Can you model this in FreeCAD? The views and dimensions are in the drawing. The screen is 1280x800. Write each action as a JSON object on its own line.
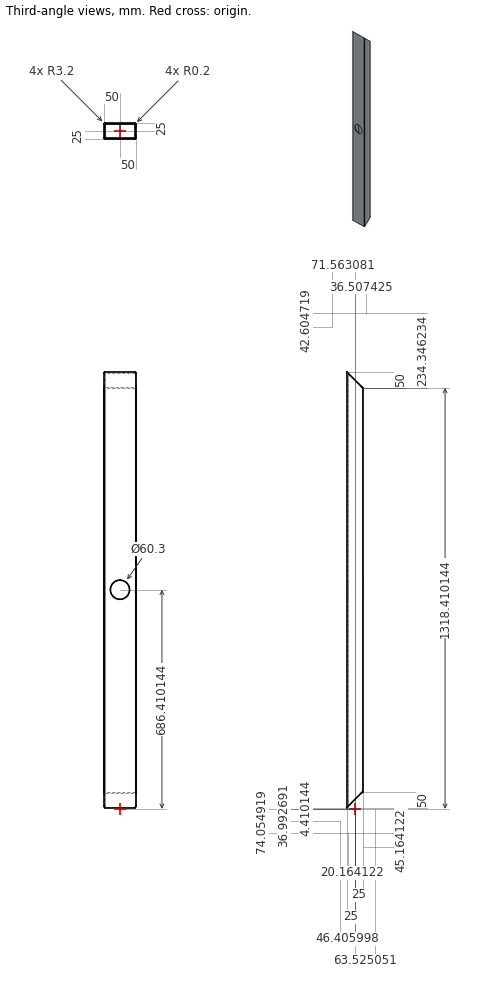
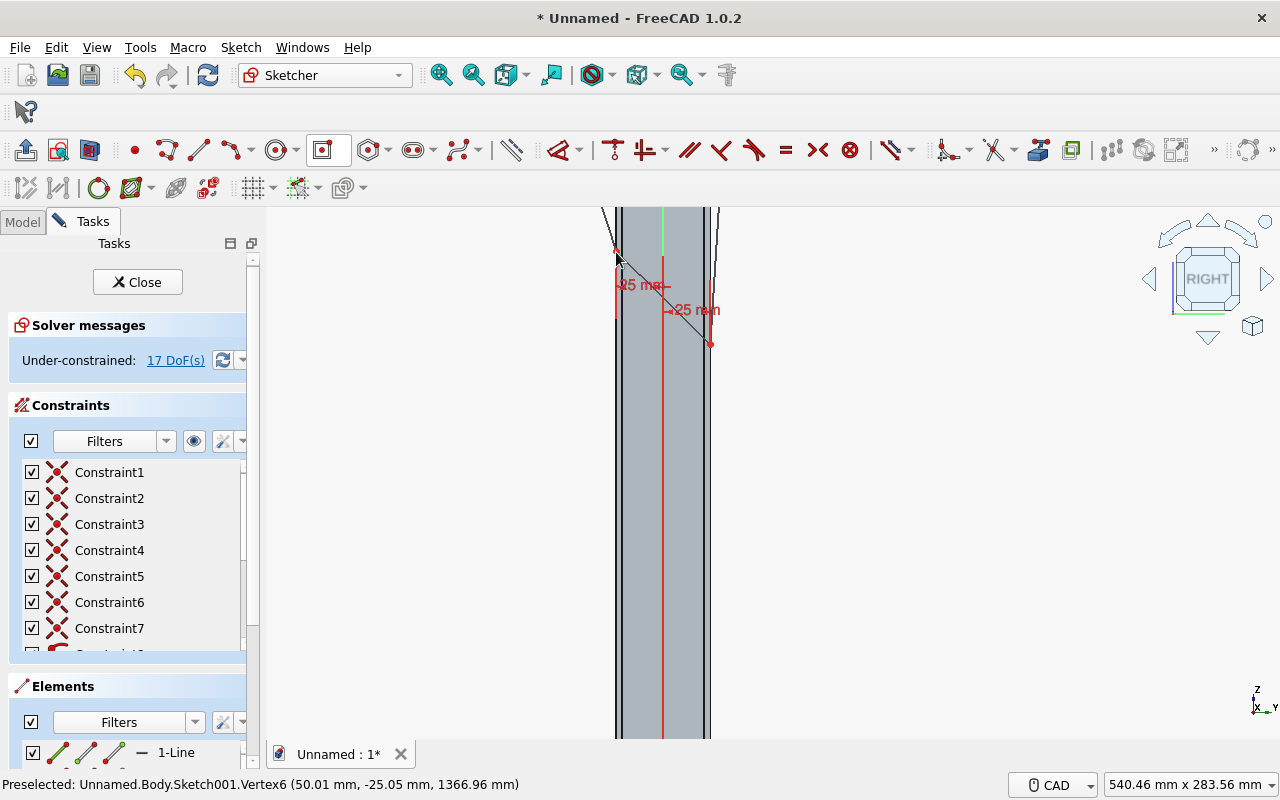
{"action": "scroll", "coordinate": [711, 349], "scroll_direction": "down", "scroll_amount": 11}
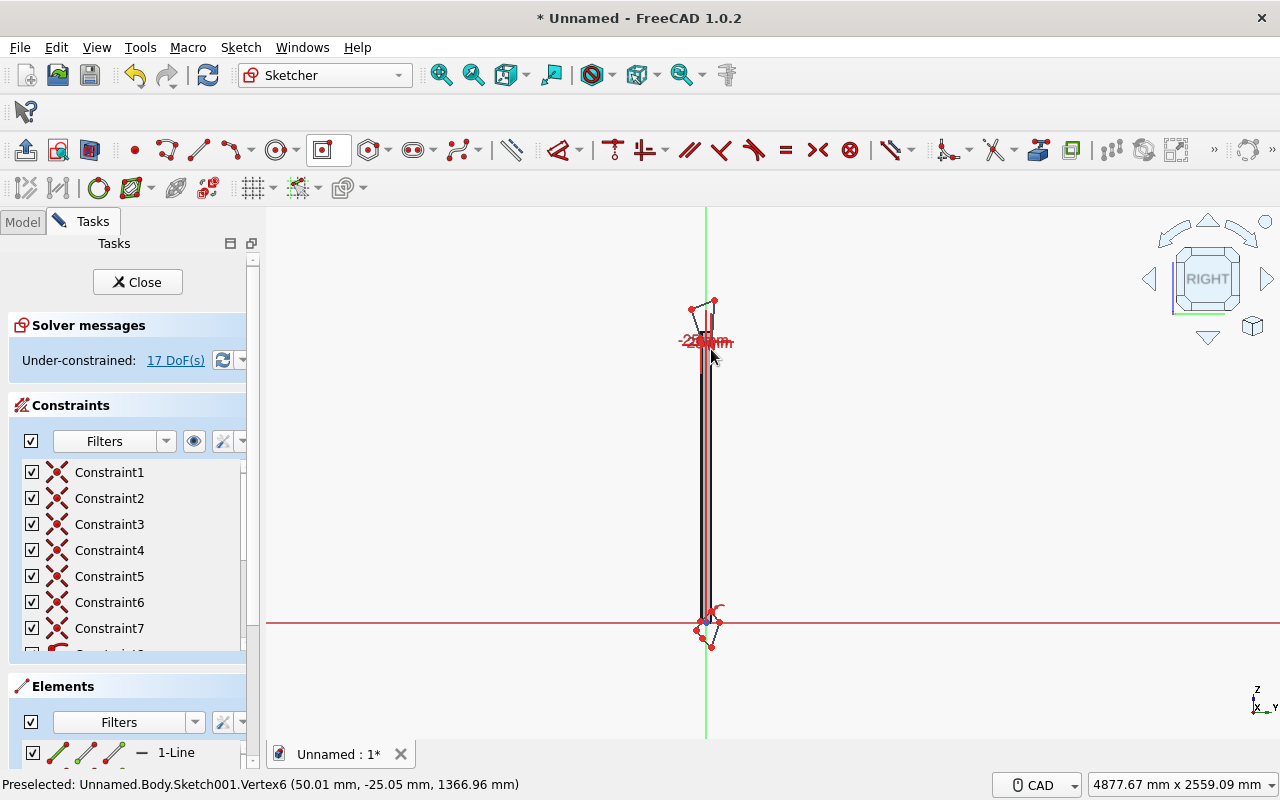
{"action": "scroll", "coordinate": [701, 622], "scroll_direction": "up", "scroll_amount": 11}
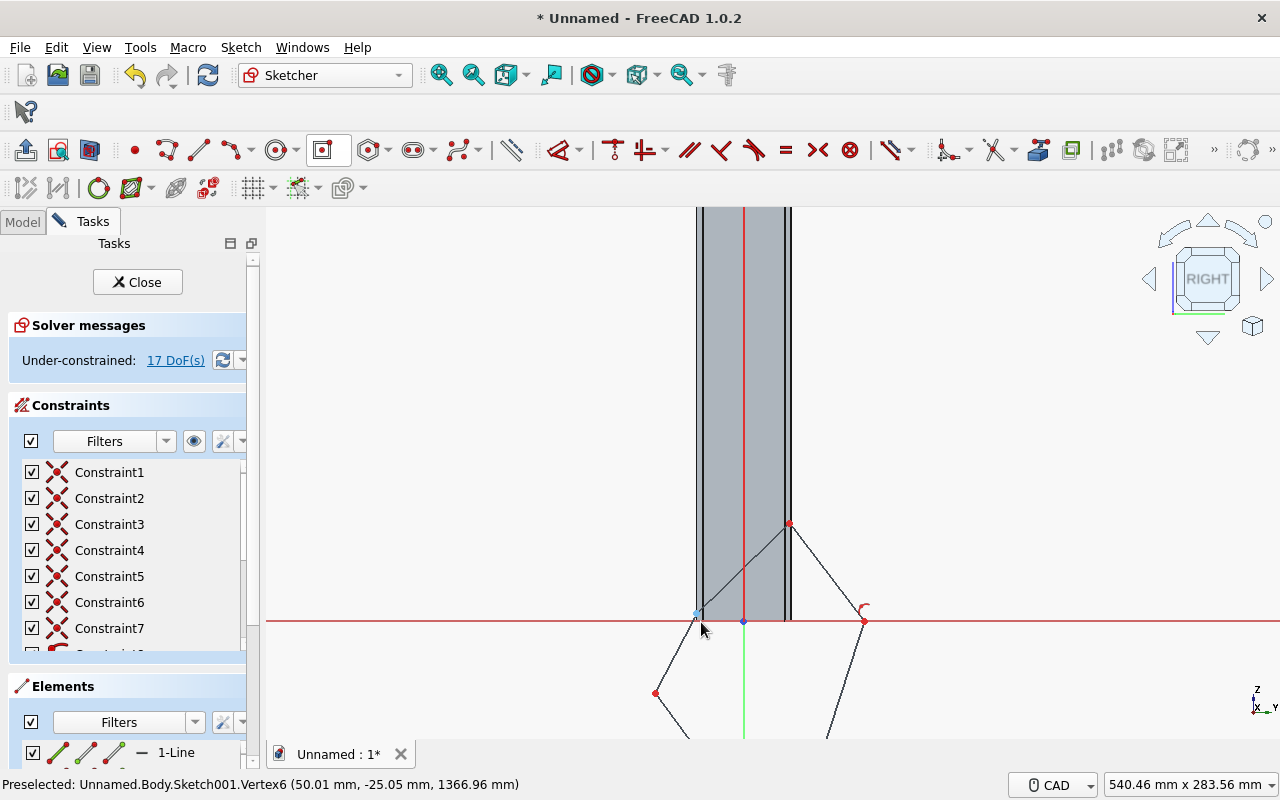
{"action": "left_click", "coordinate": [697, 614]}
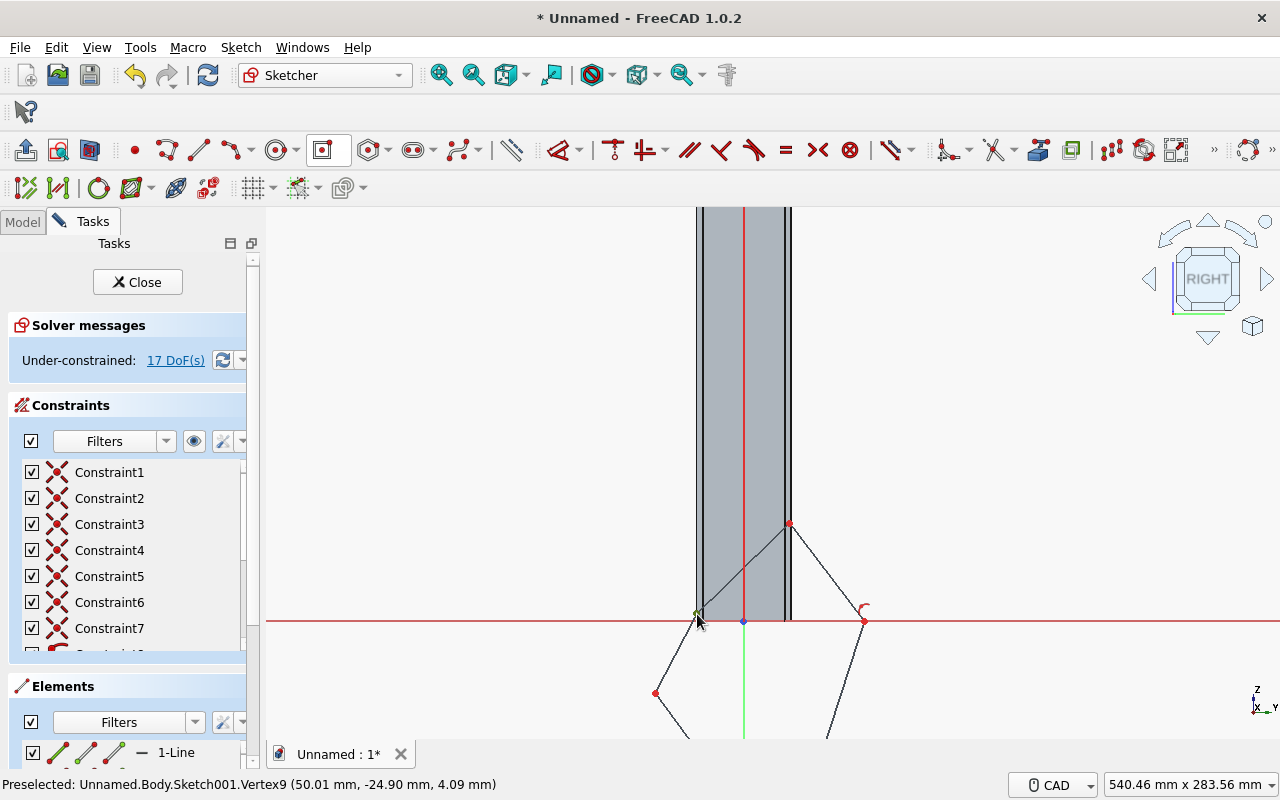
{"action": "left_click", "coordinate": [582, 150]}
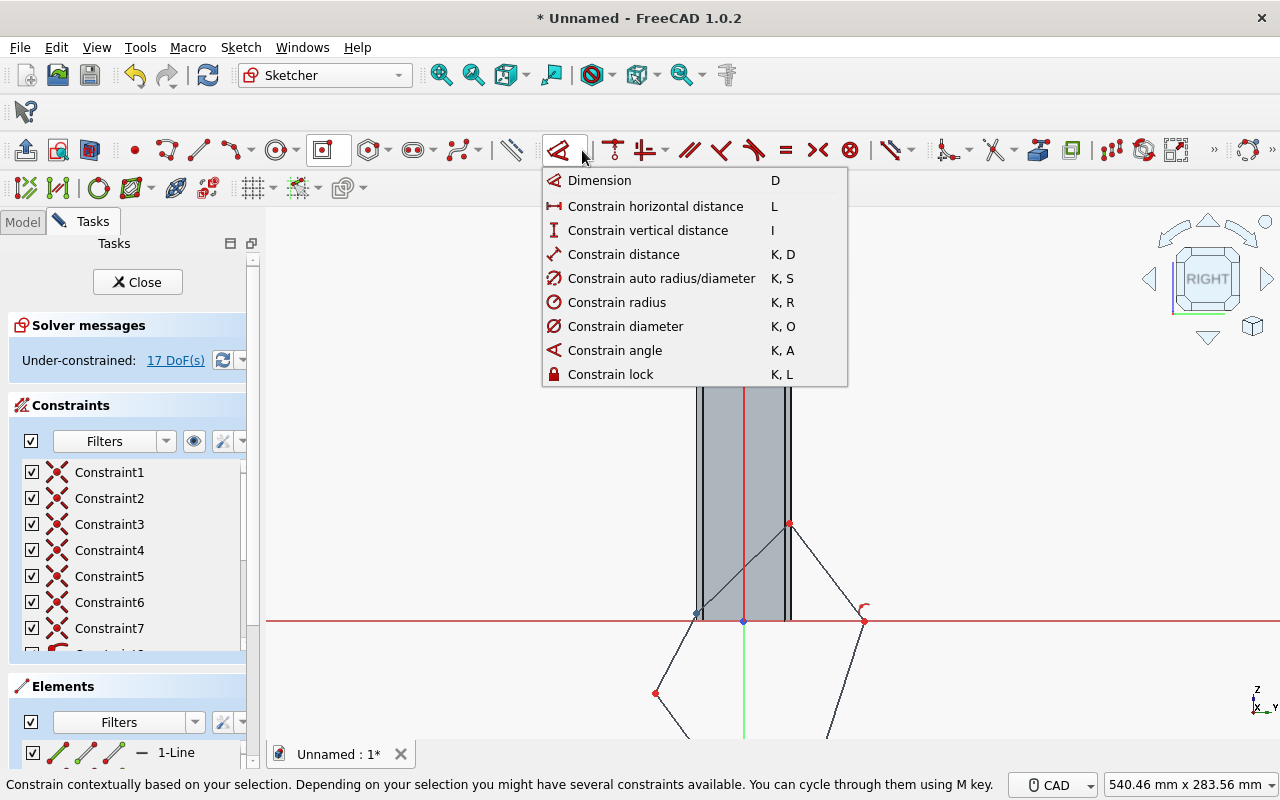
{"action": "left_click", "coordinate": [695, 206]}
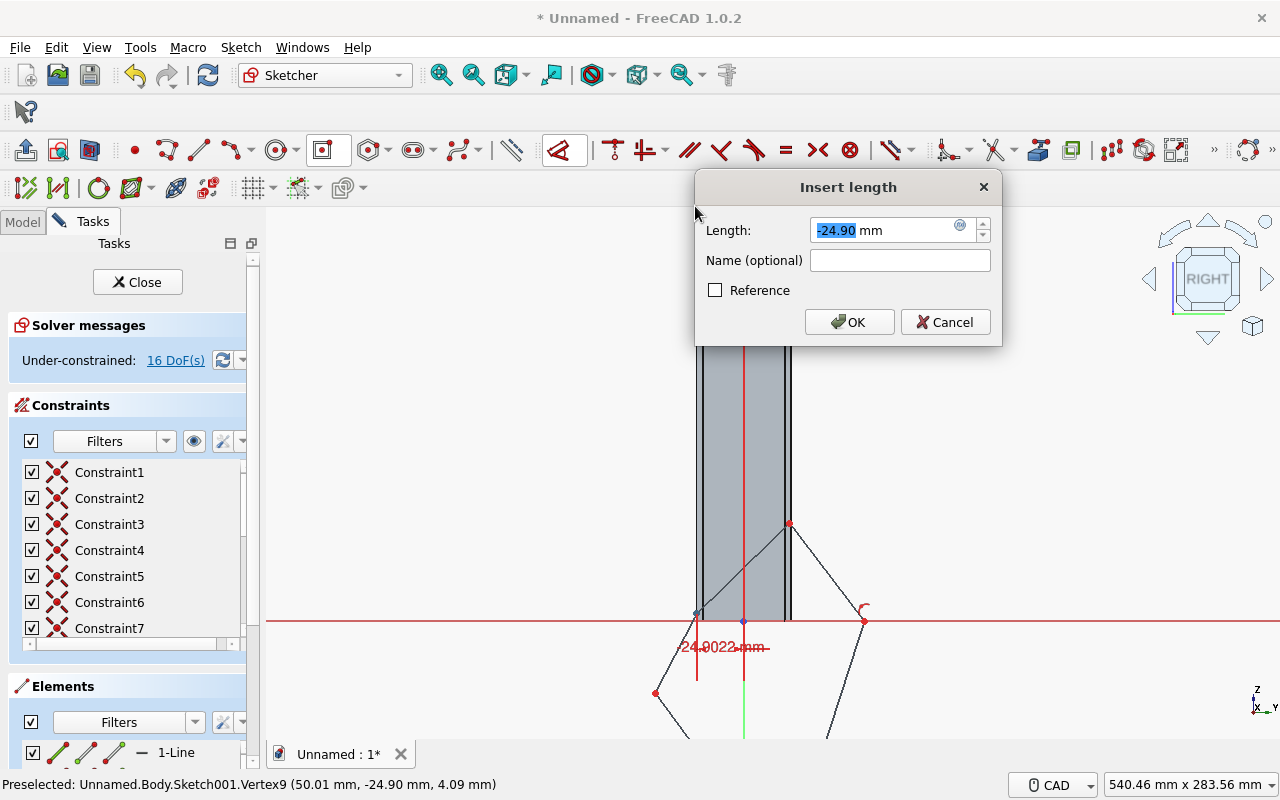
{"action": "type", "text": "-25"}
{"action": "key", "text": "Return"}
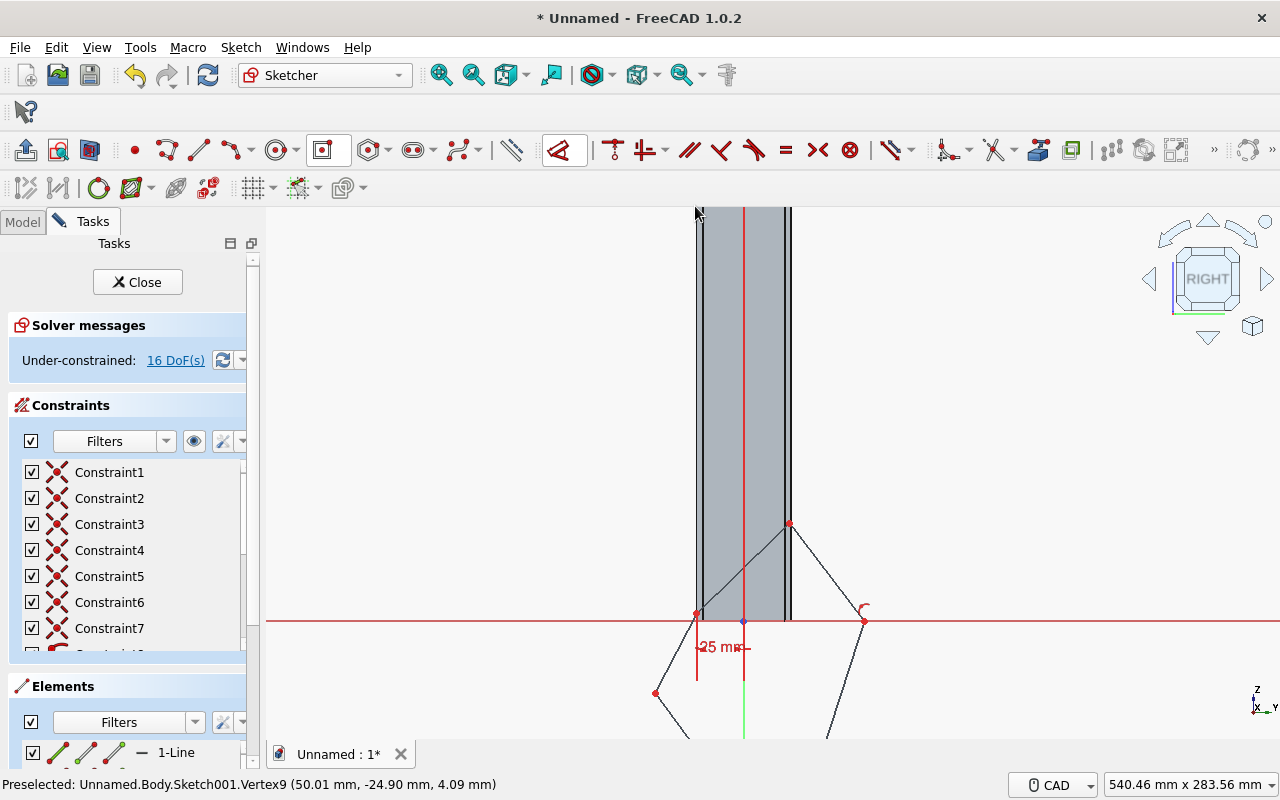
{"action": "scroll", "coordinate": [701, 622], "scroll_direction": "down", "scroll_amount": 11}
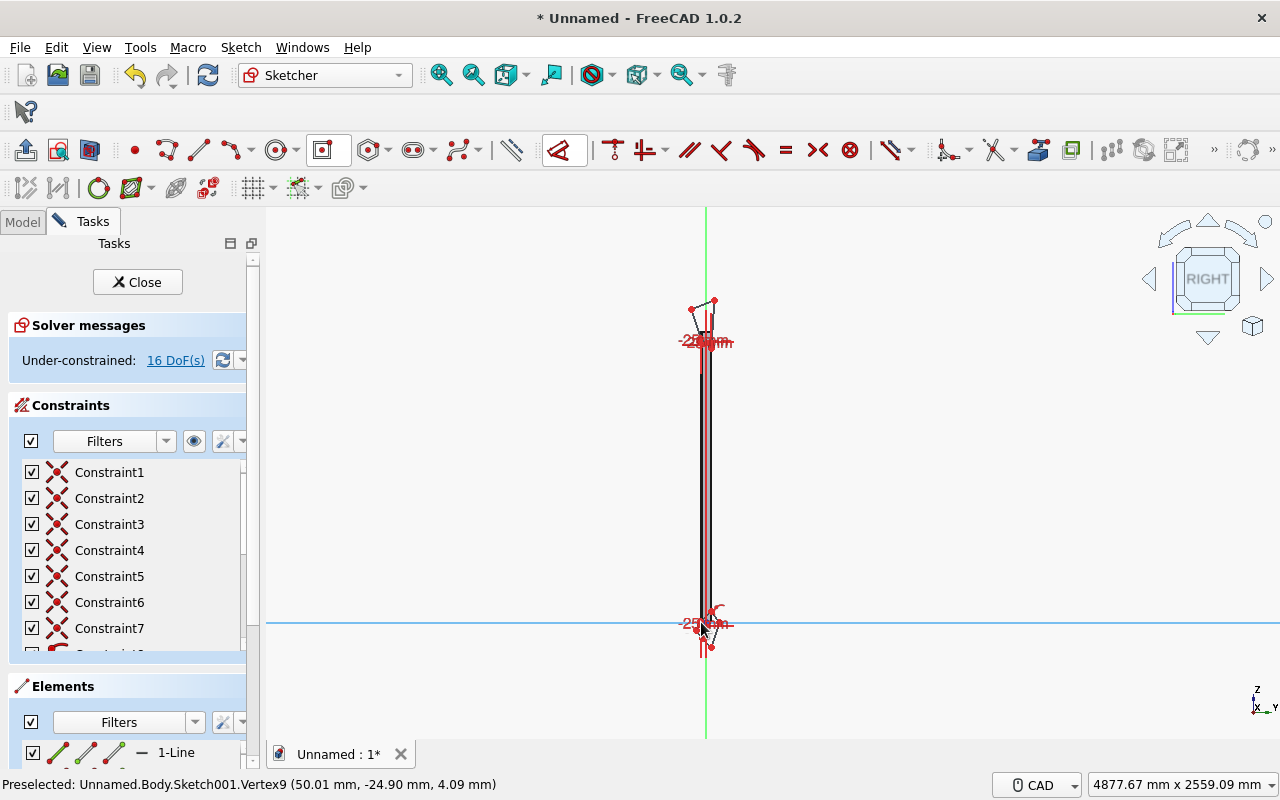
{"action": "scroll", "coordinate": [711, 648], "scroll_direction": "up", "scroll_amount": 11}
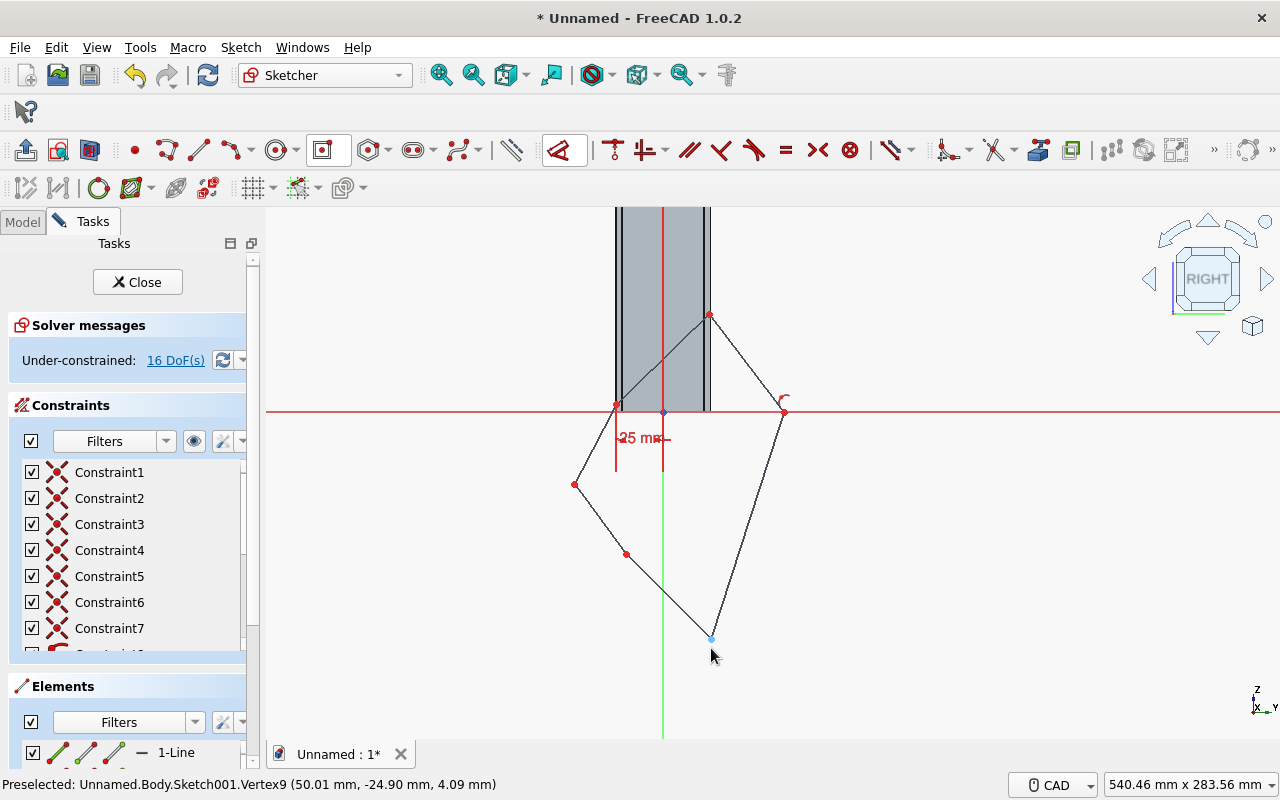
{"action": "left_click", "coordinate": [711, 639]}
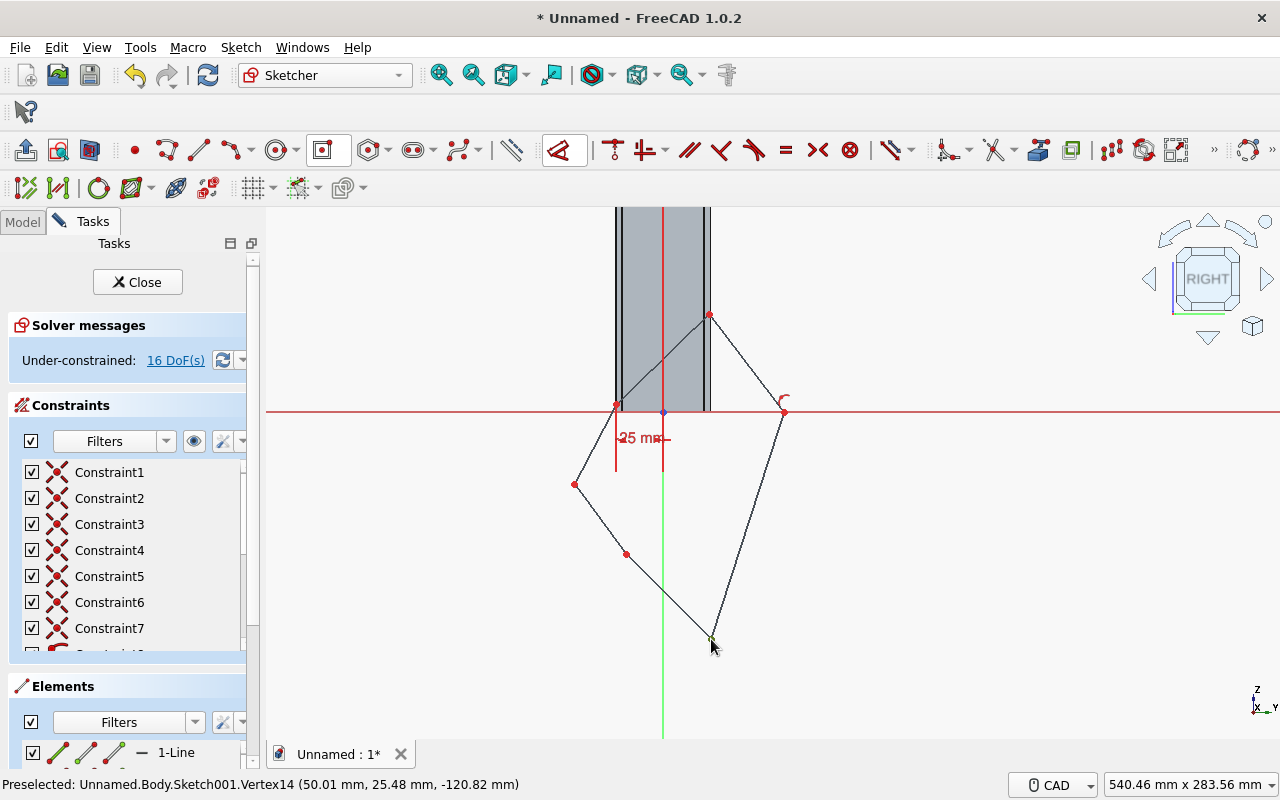
{"action": "left_click", "coordinate": [582, 150]}